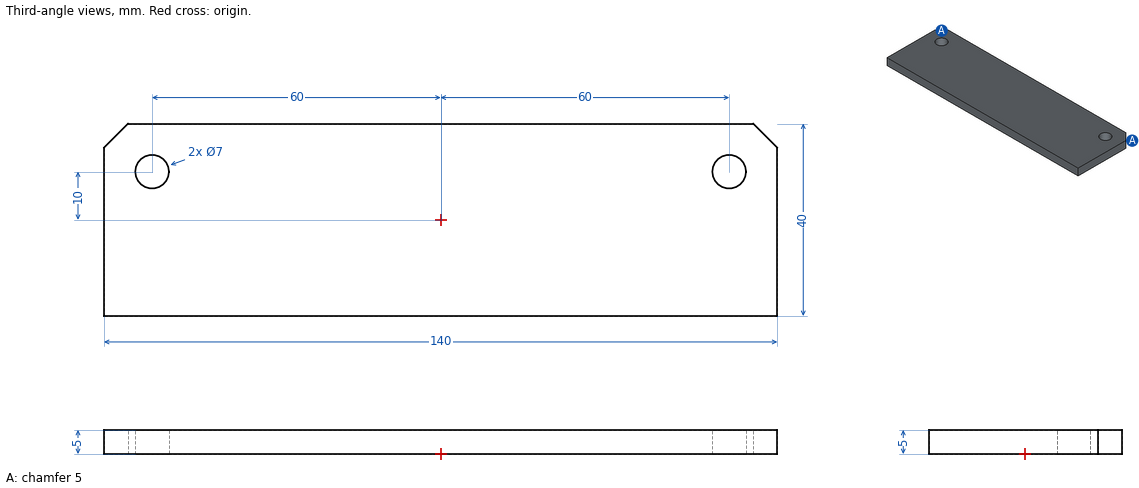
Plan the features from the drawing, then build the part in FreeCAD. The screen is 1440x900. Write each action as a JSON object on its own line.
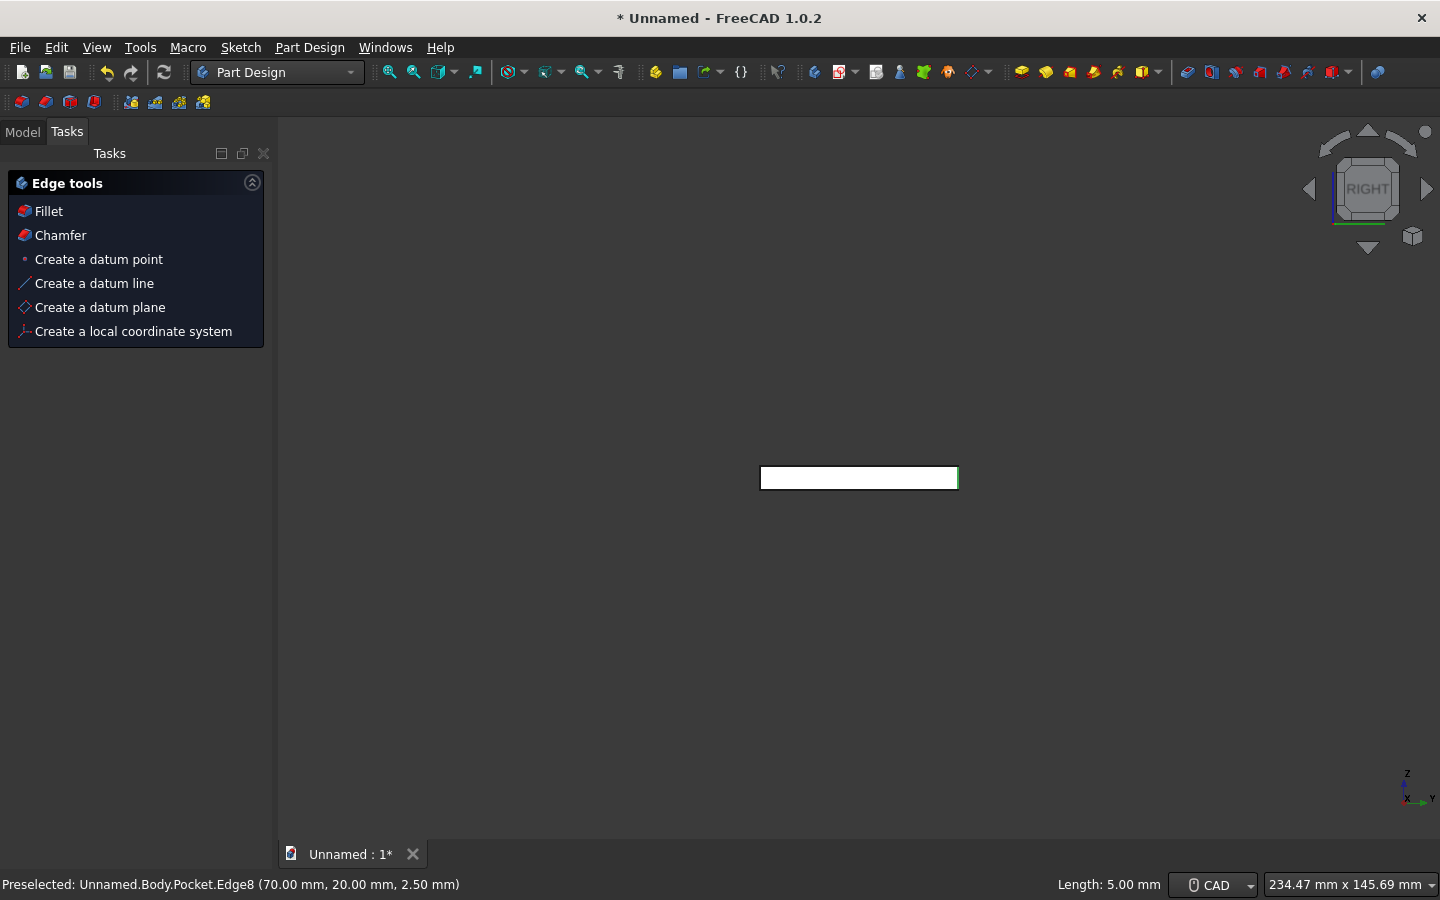
{"action": "key", "text": "5"}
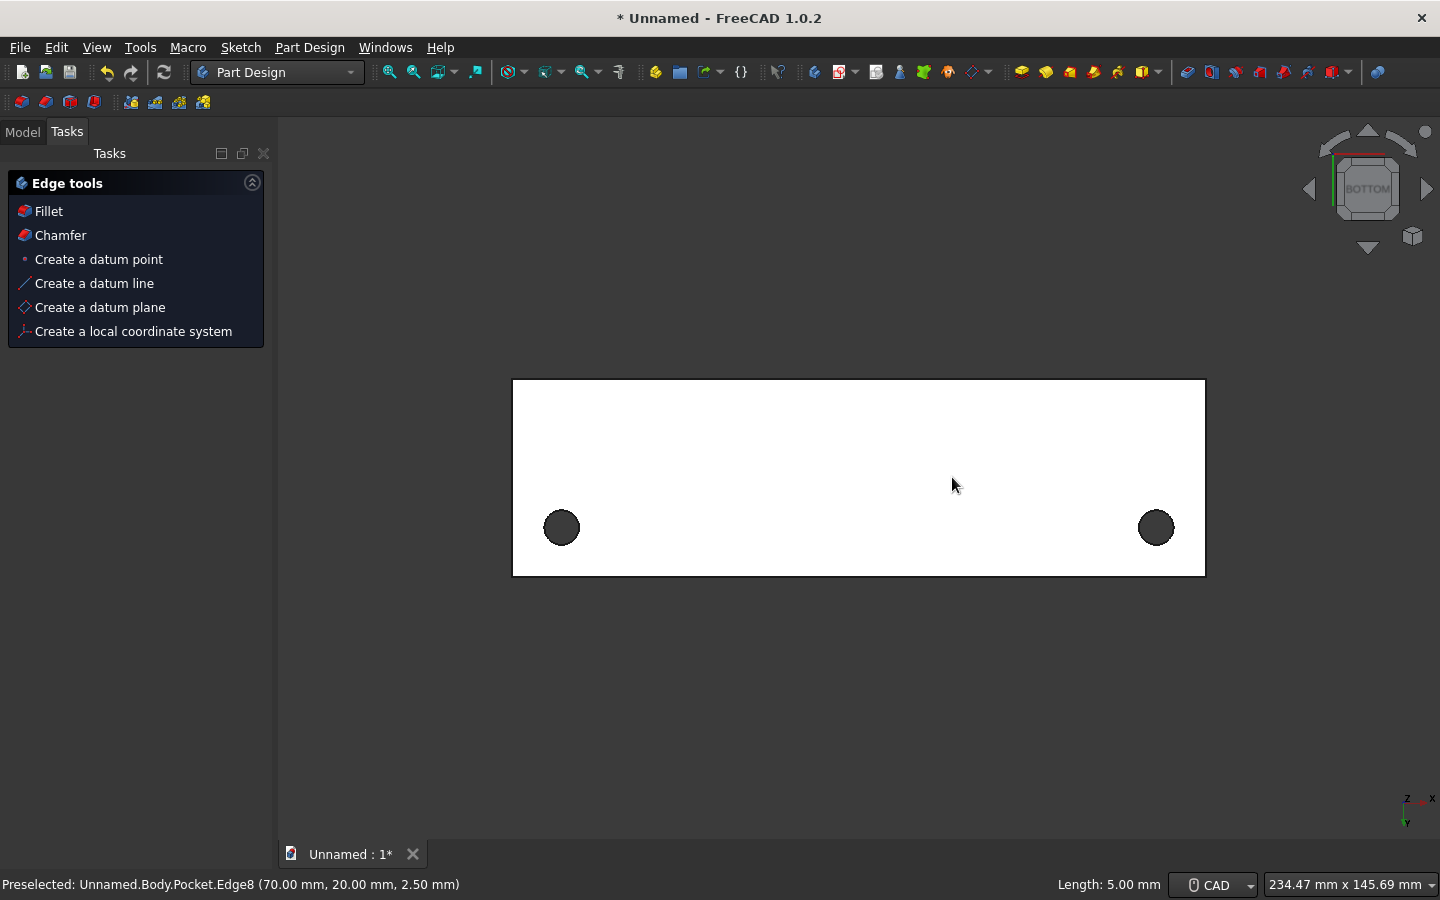
{"action": "key", "text": "4"}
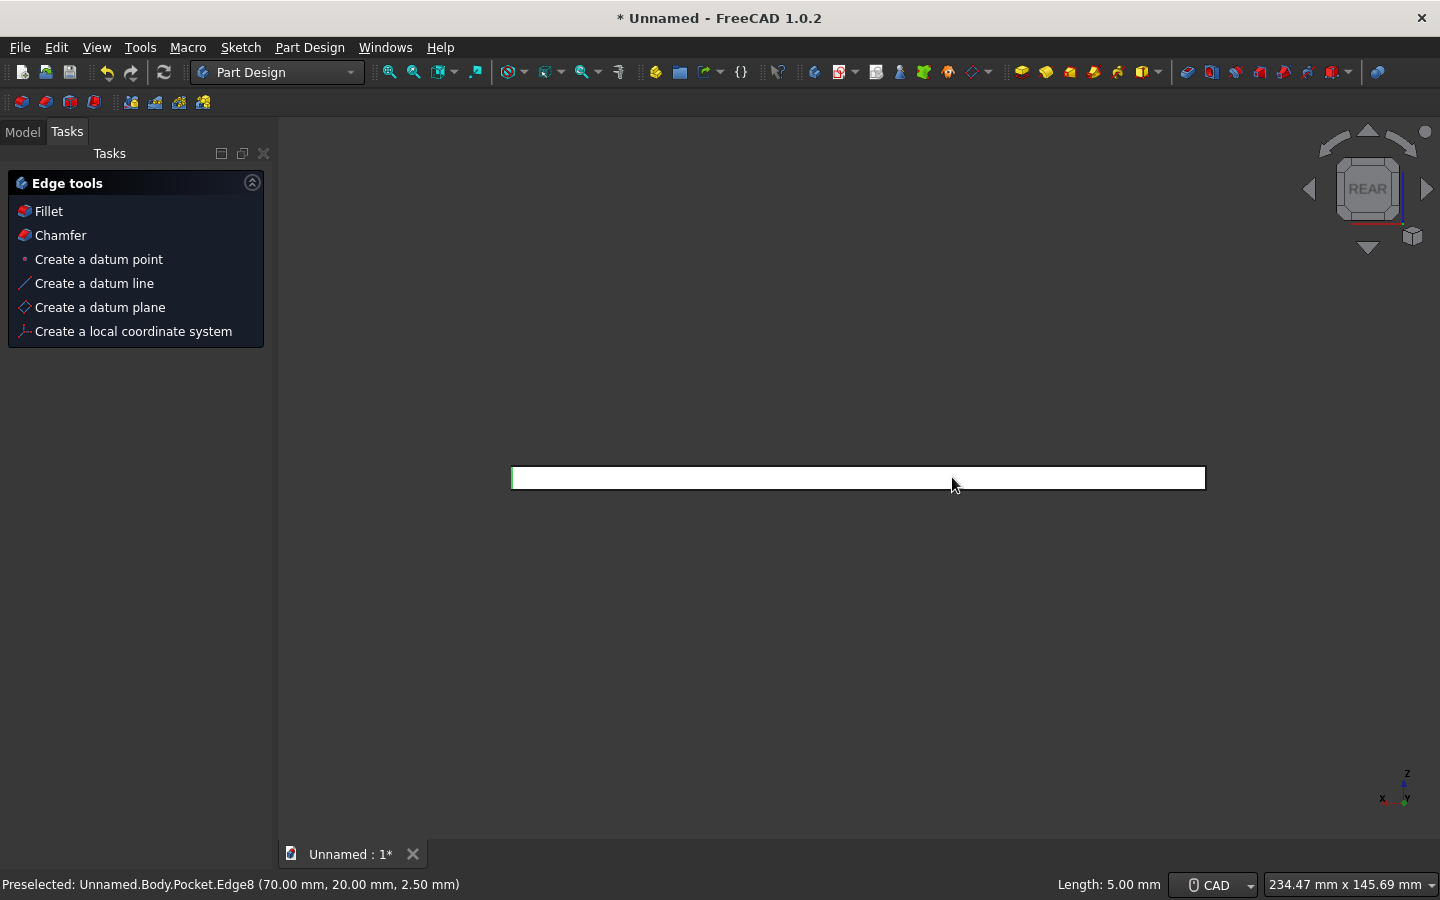
{"action": "left_click", "coordinate": [1206, 477], "text": "ctrl"}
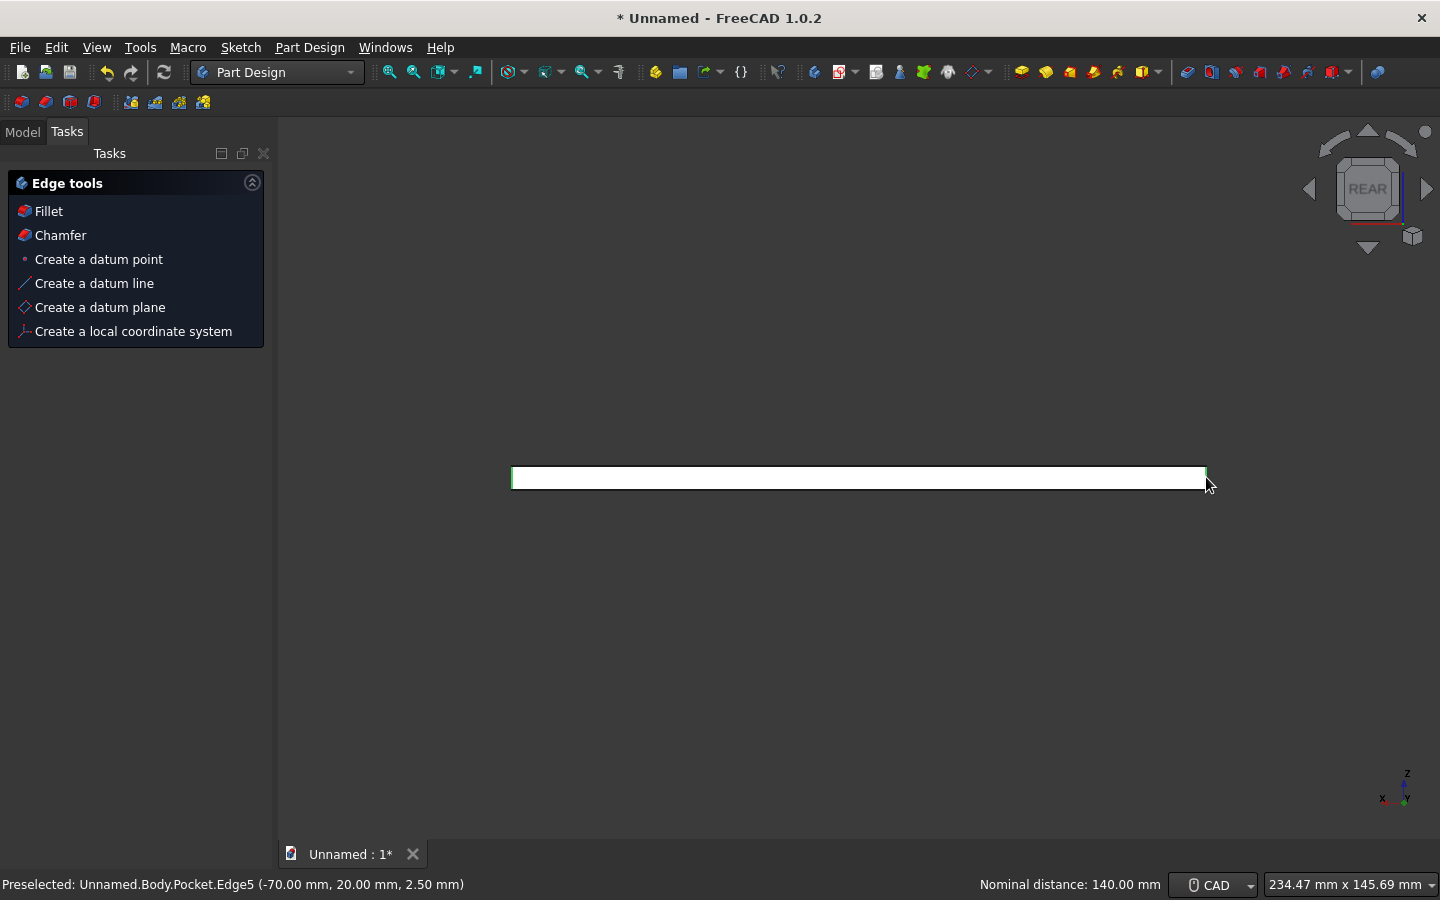
{"action": "left_click", "coordinate": [46, 102]}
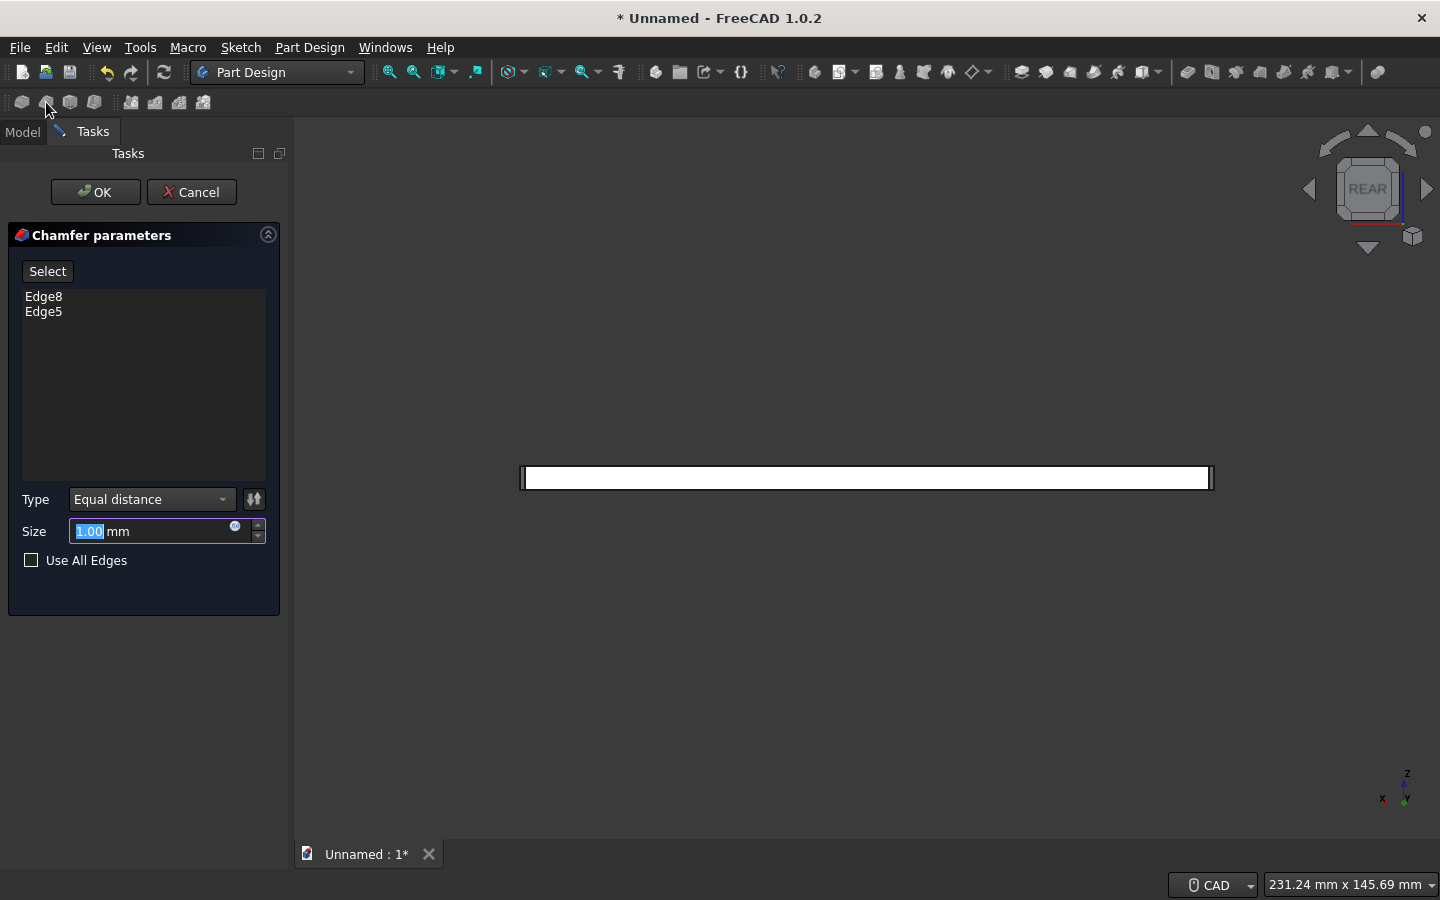
{"action": "type", "text": "5"}
{"action": "key", "text": "Tab"}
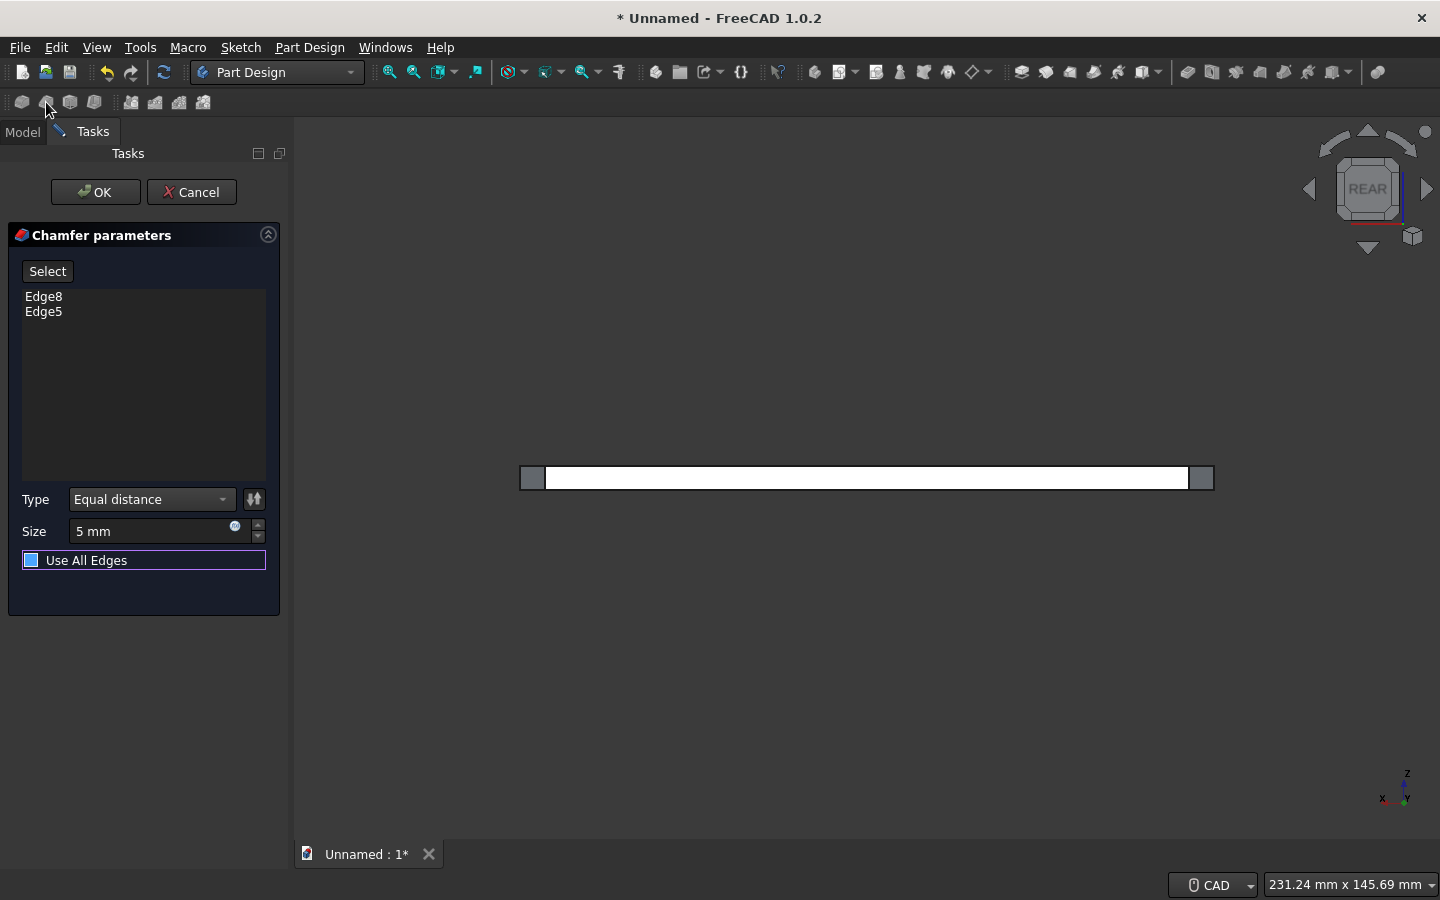
{"action": "left_click", "coordinate": [96, 192]}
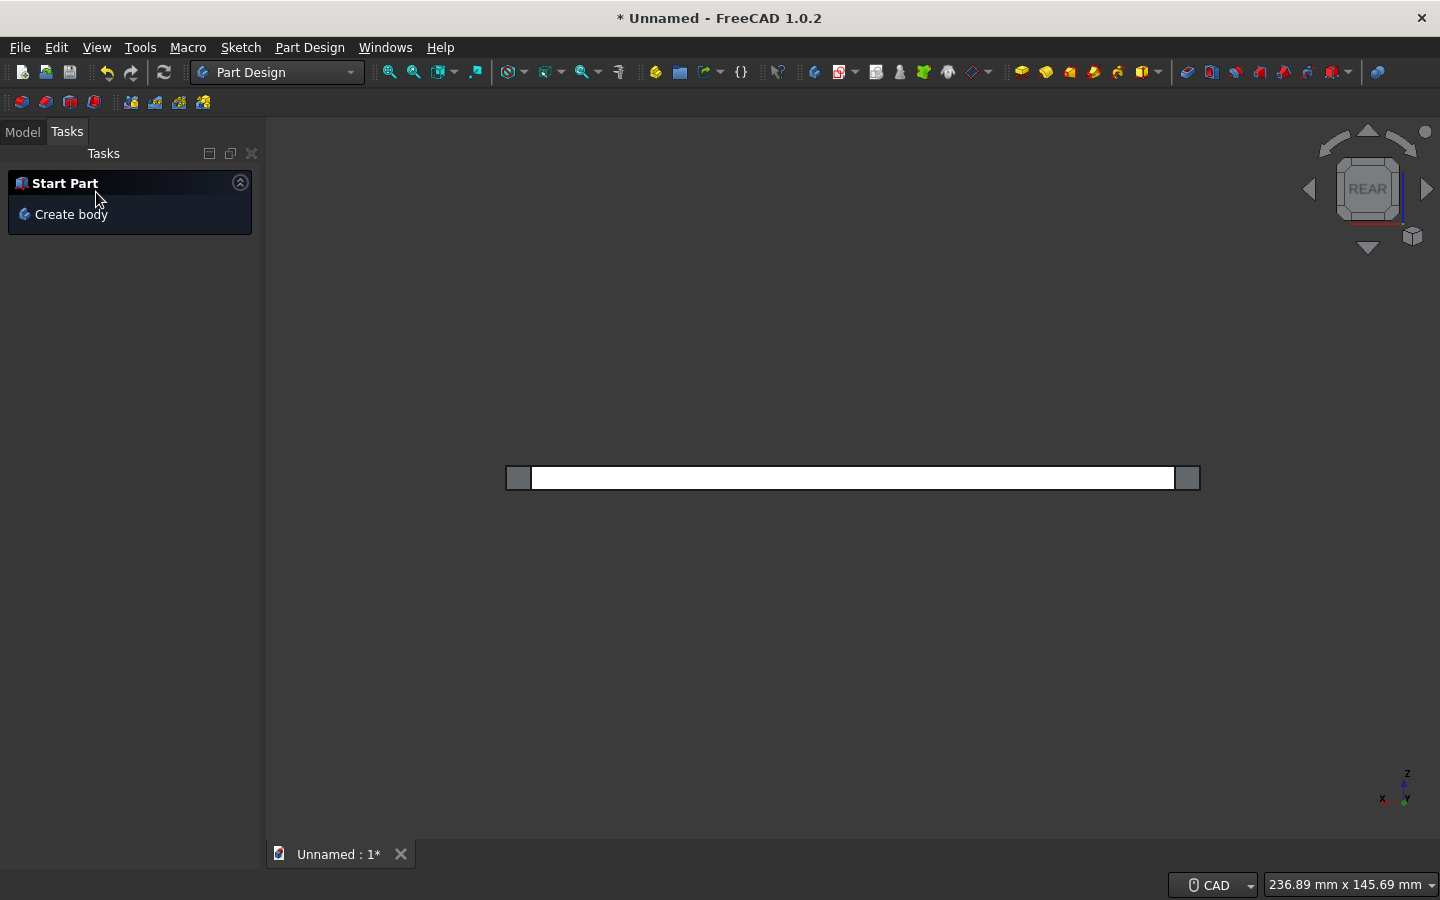
{"action": "key", "text": "0"}